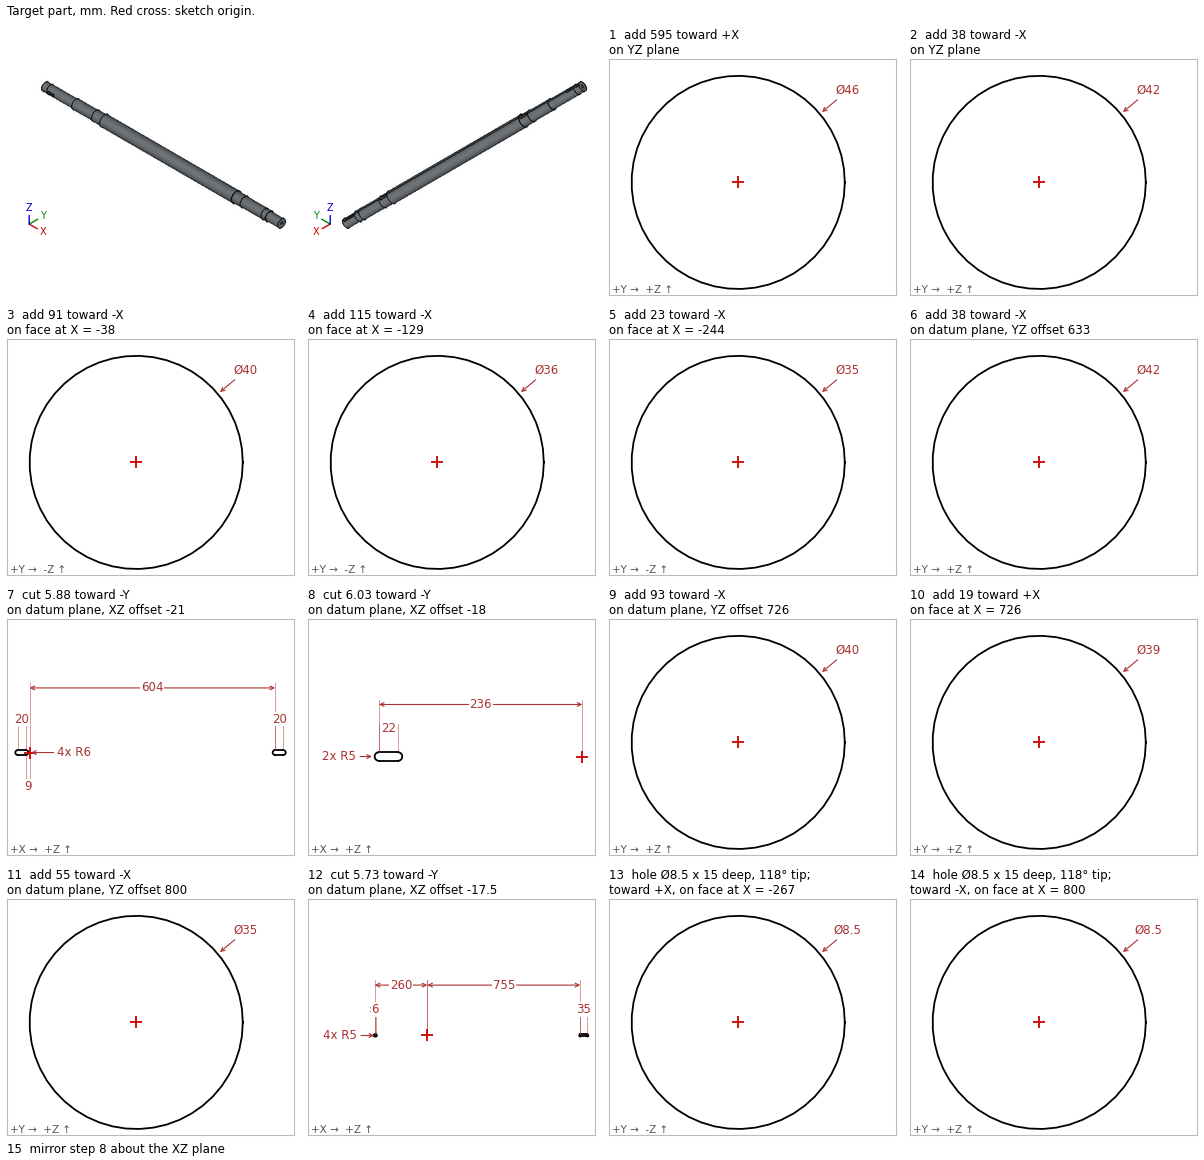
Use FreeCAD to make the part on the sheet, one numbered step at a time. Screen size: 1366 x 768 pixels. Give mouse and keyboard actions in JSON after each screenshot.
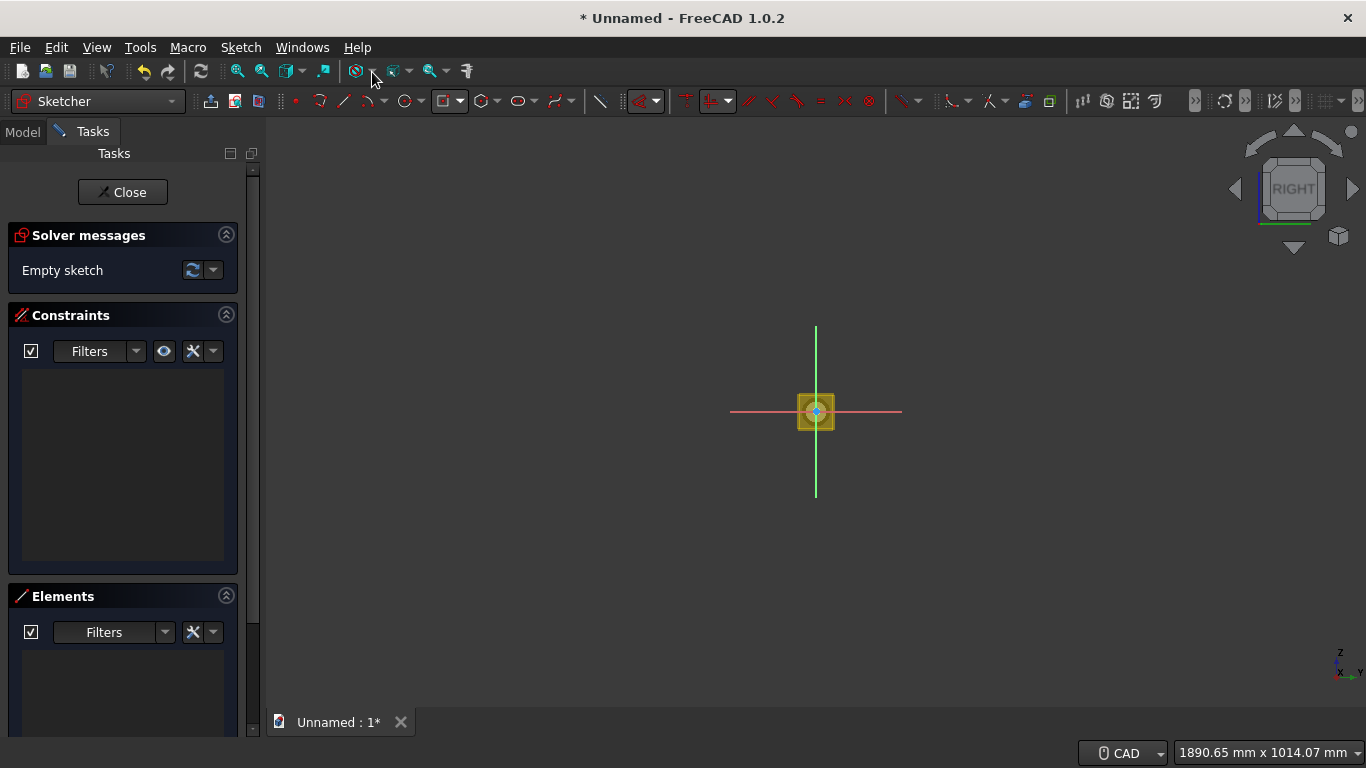
{"action": "scroll", "coordinate": [820, 412], "scroll_direction": "up", "scroll_amount": 15}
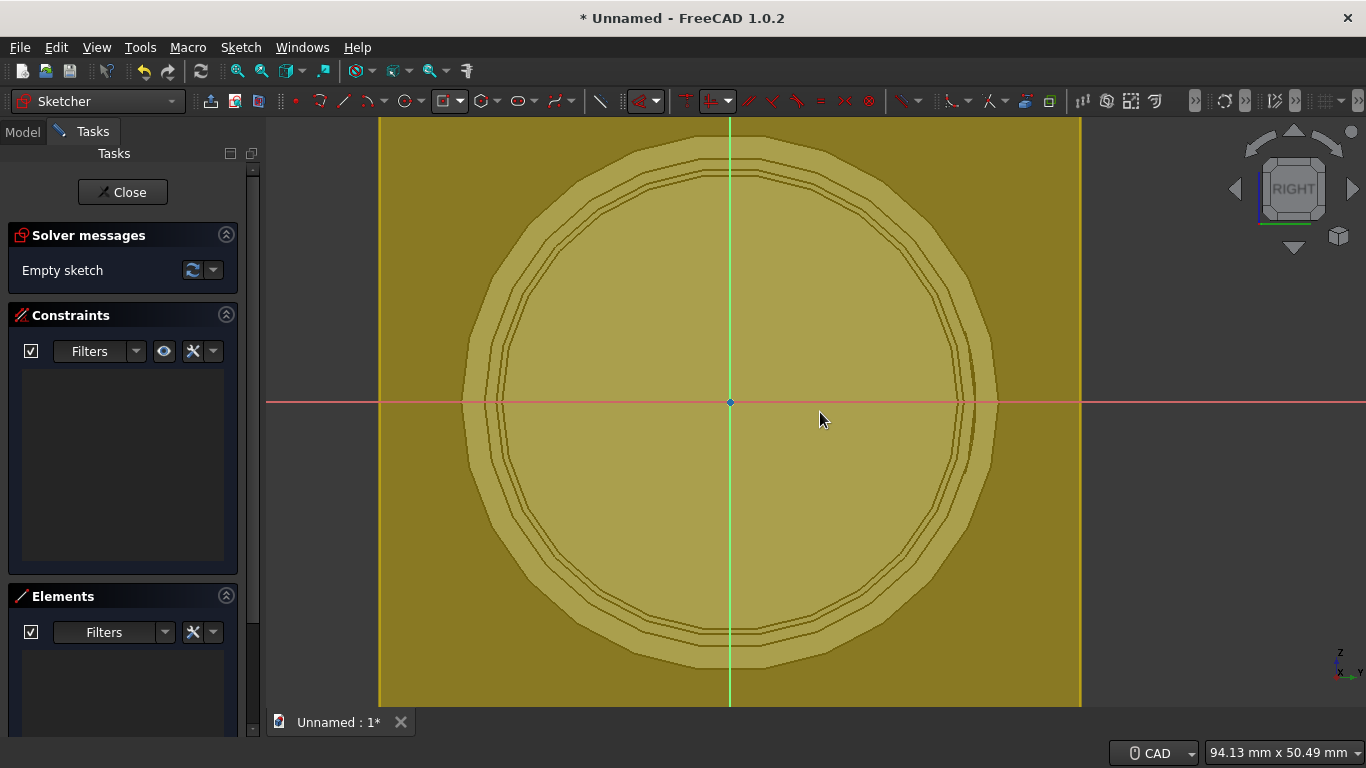
{"action": "left_click", "coordinate": [406, 102]}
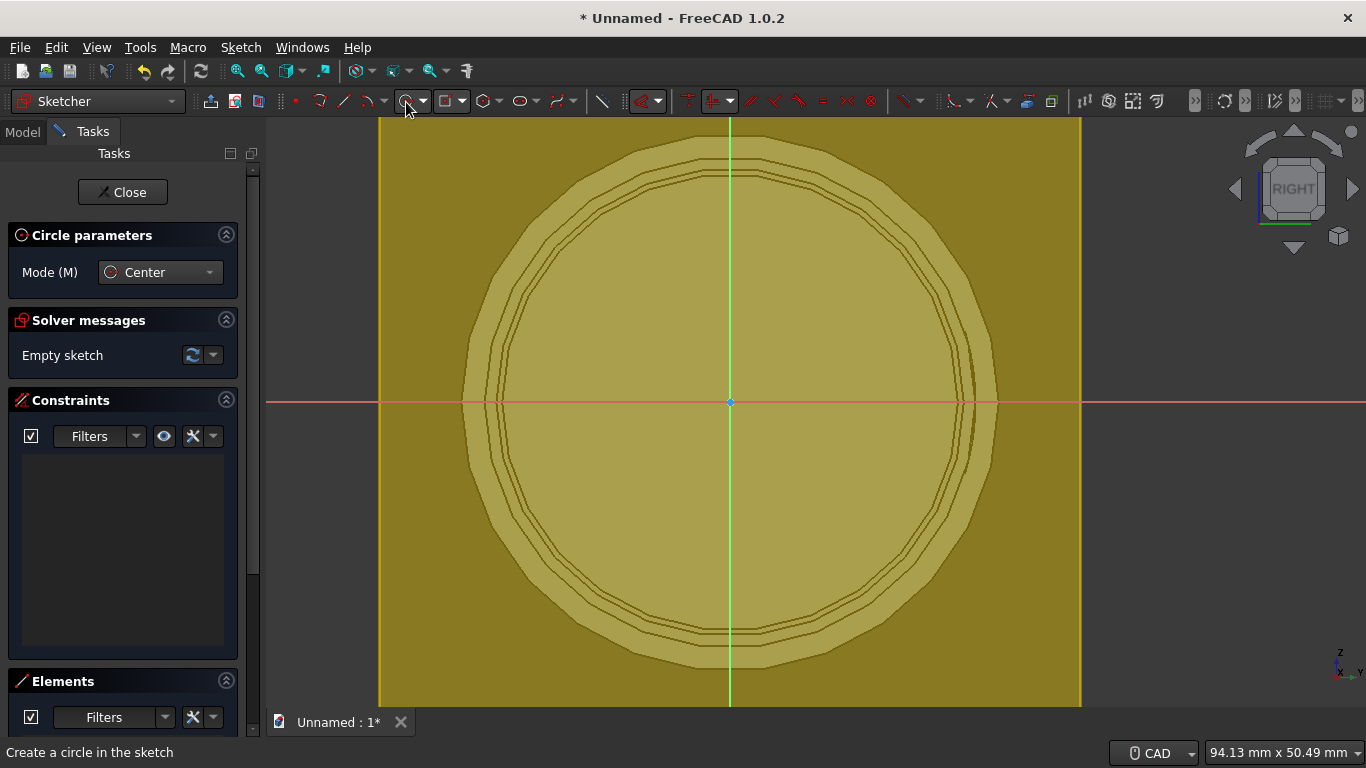
{"action": "left_click", "coordinate": [730, 402]}
{"action": "mouse_move", "coordinate": [875, 258]}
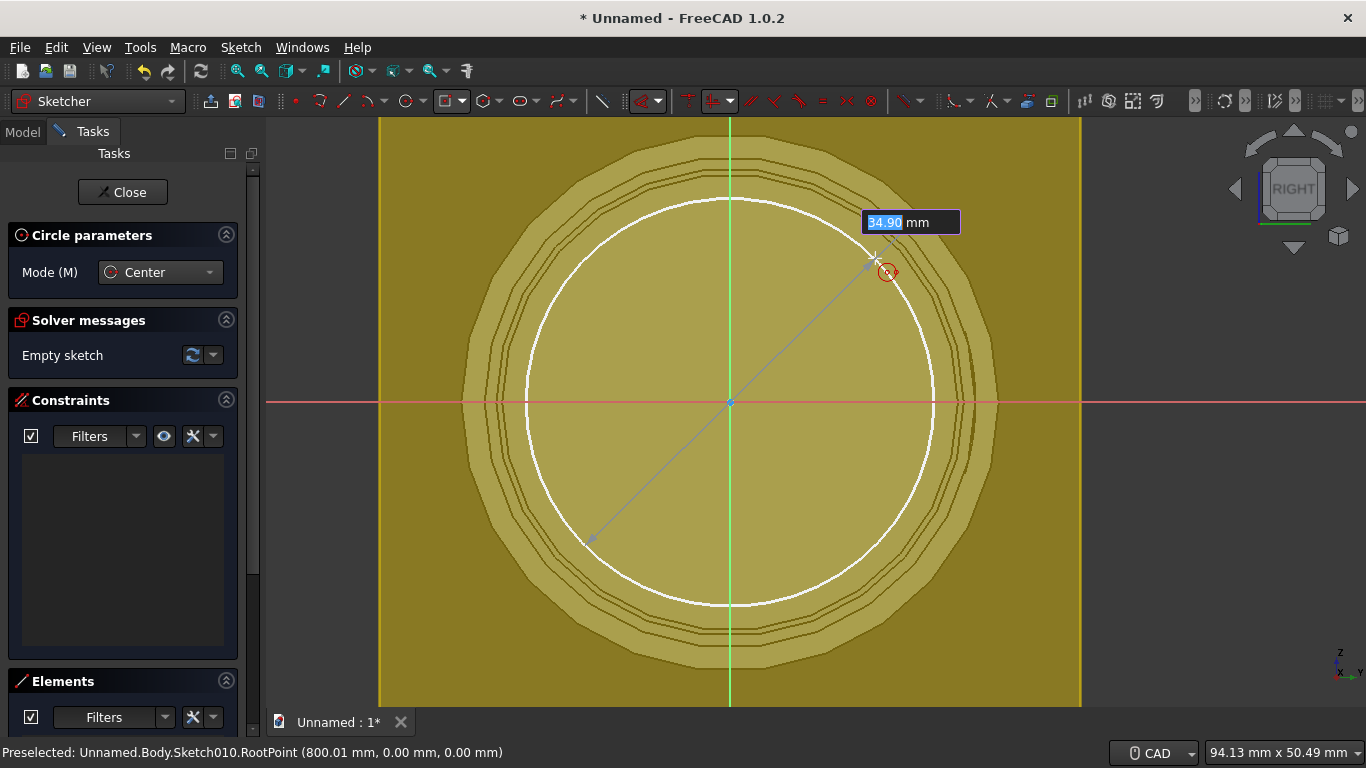
{"action": "type", "text": "35"}
{"action": "key", "text": "Return"}
{"action": "key", "text": "Escape"}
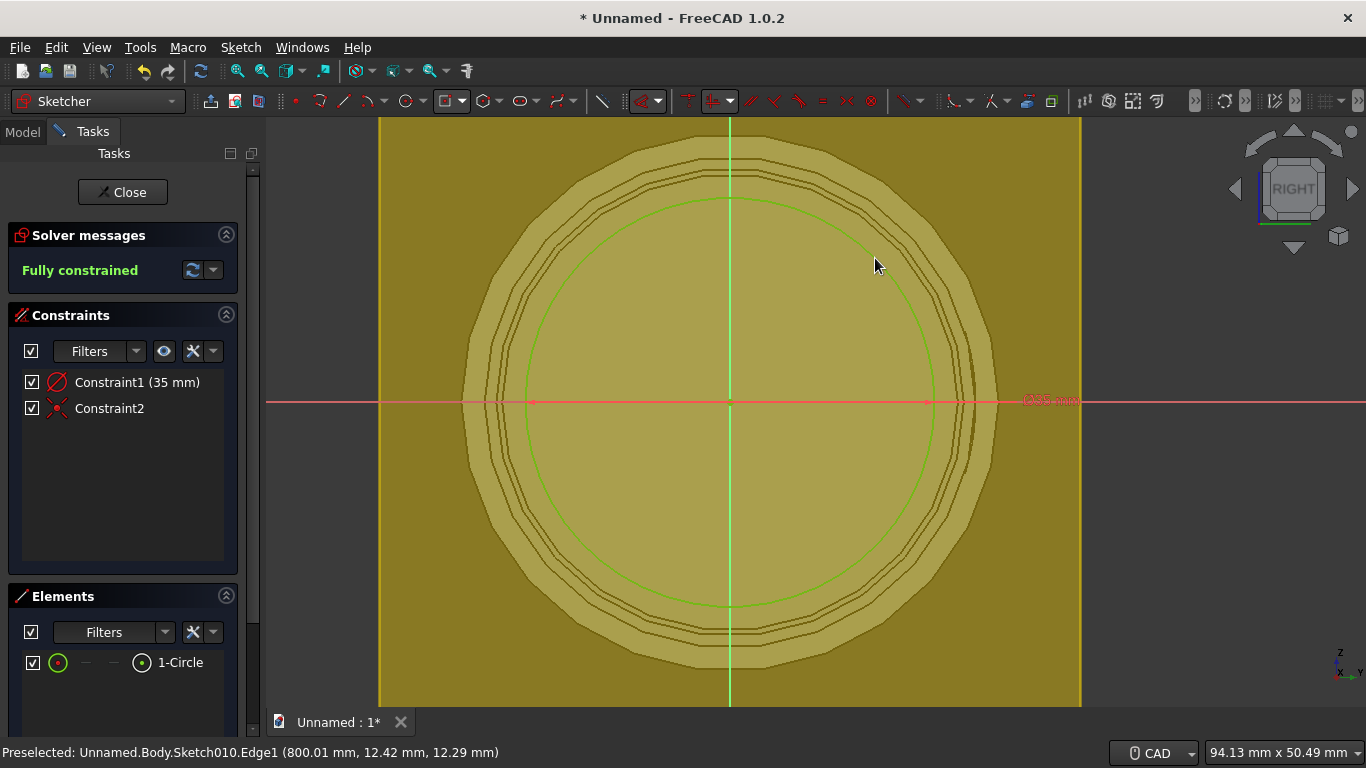
{"action": "left_click", "coordinate": [123, 192]}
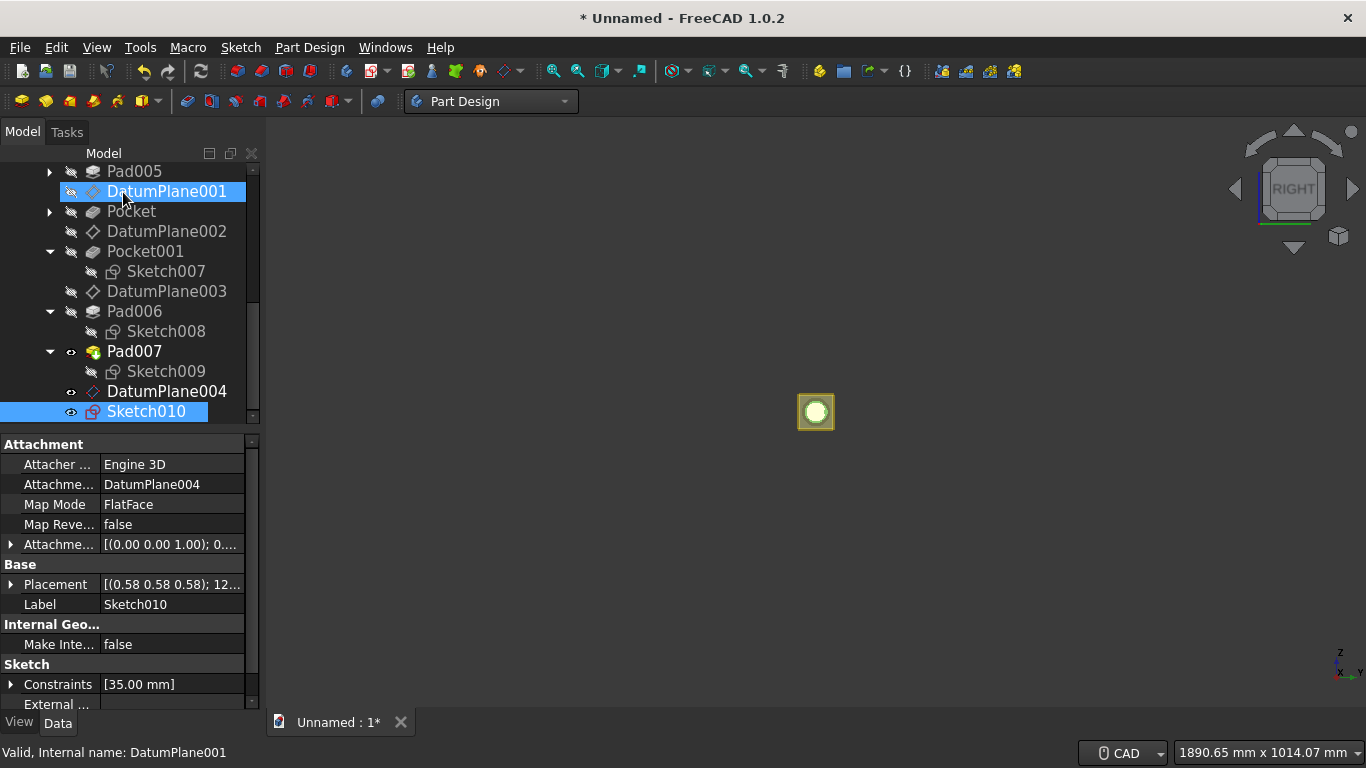
{"action": "left_click", "coordinate": [22, 102]}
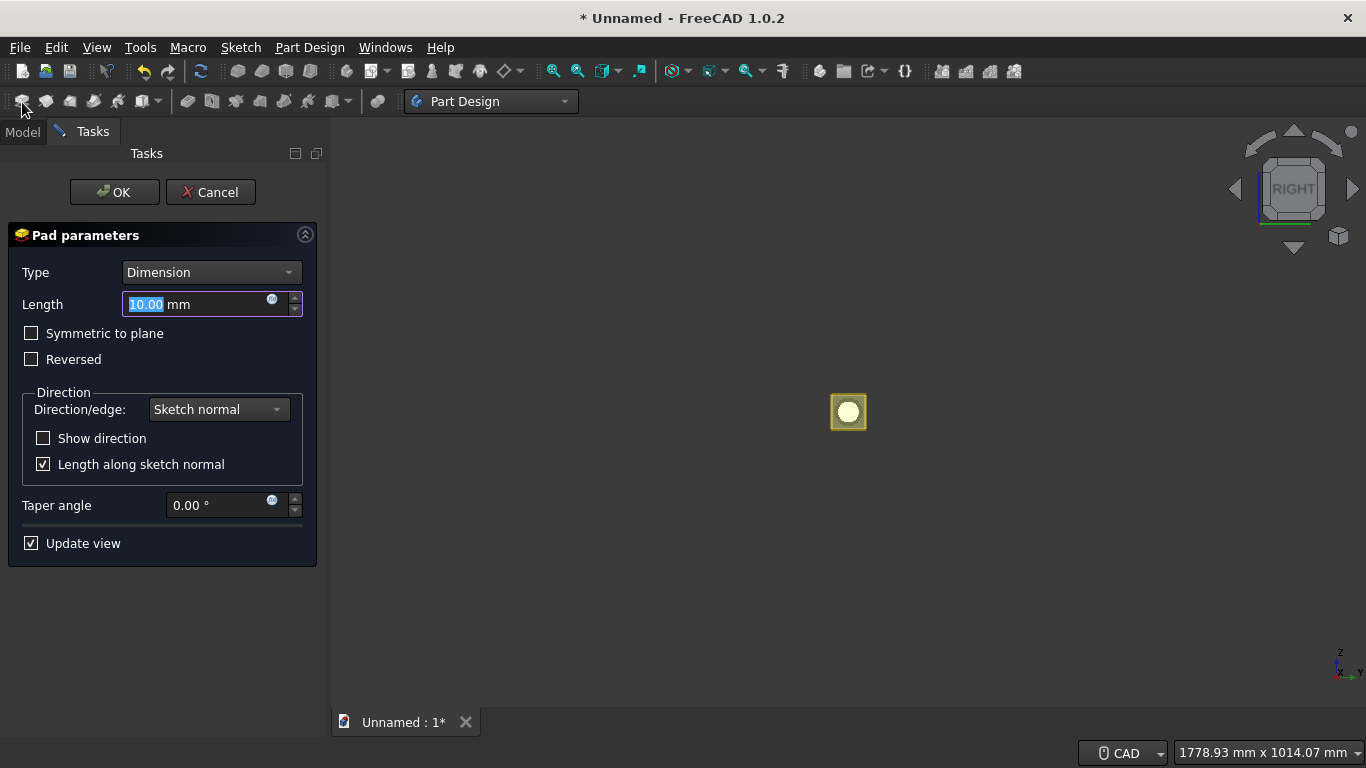
{"action": "type", "text": "55"}
{"action": "key", "text": "Tab"}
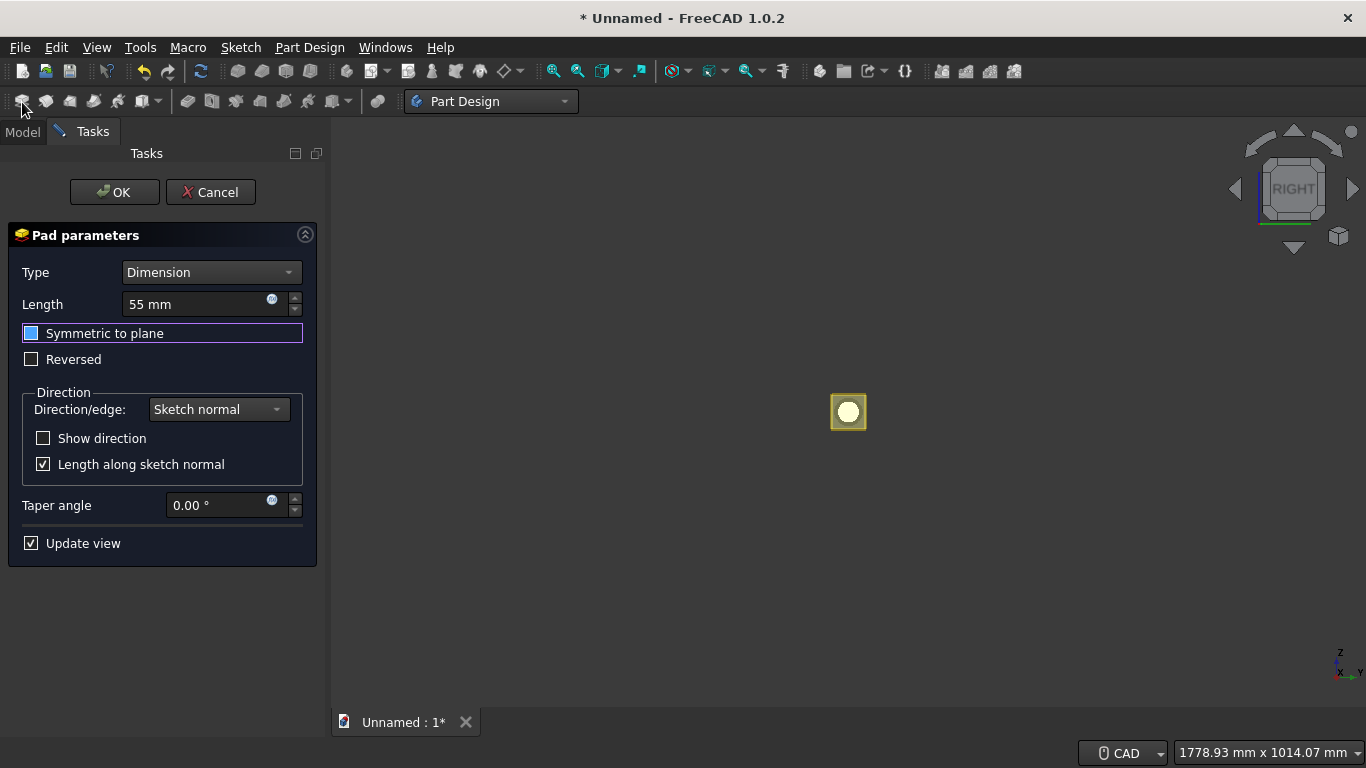
{"action": "left_click", "coordinate": [30, 359]}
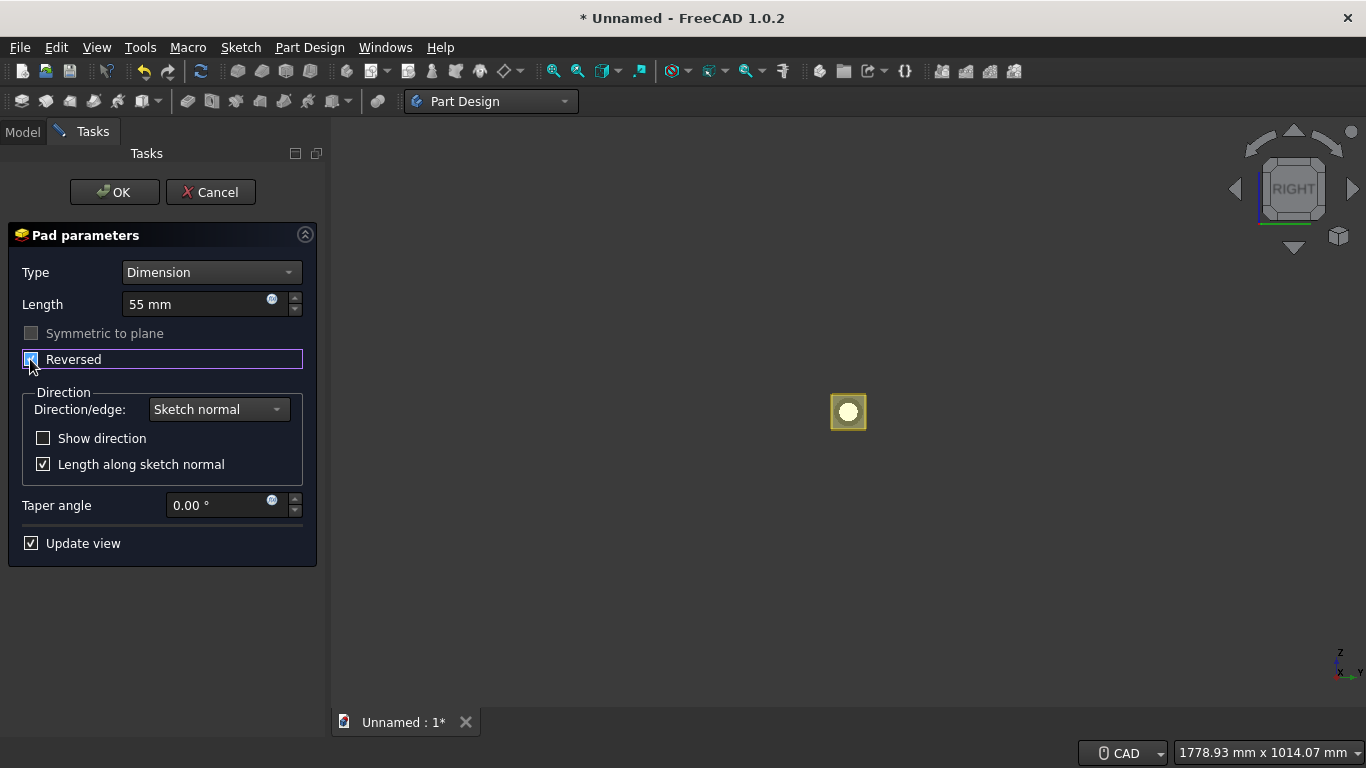
{"action": "left_click", "coordinate": [115, 192]}